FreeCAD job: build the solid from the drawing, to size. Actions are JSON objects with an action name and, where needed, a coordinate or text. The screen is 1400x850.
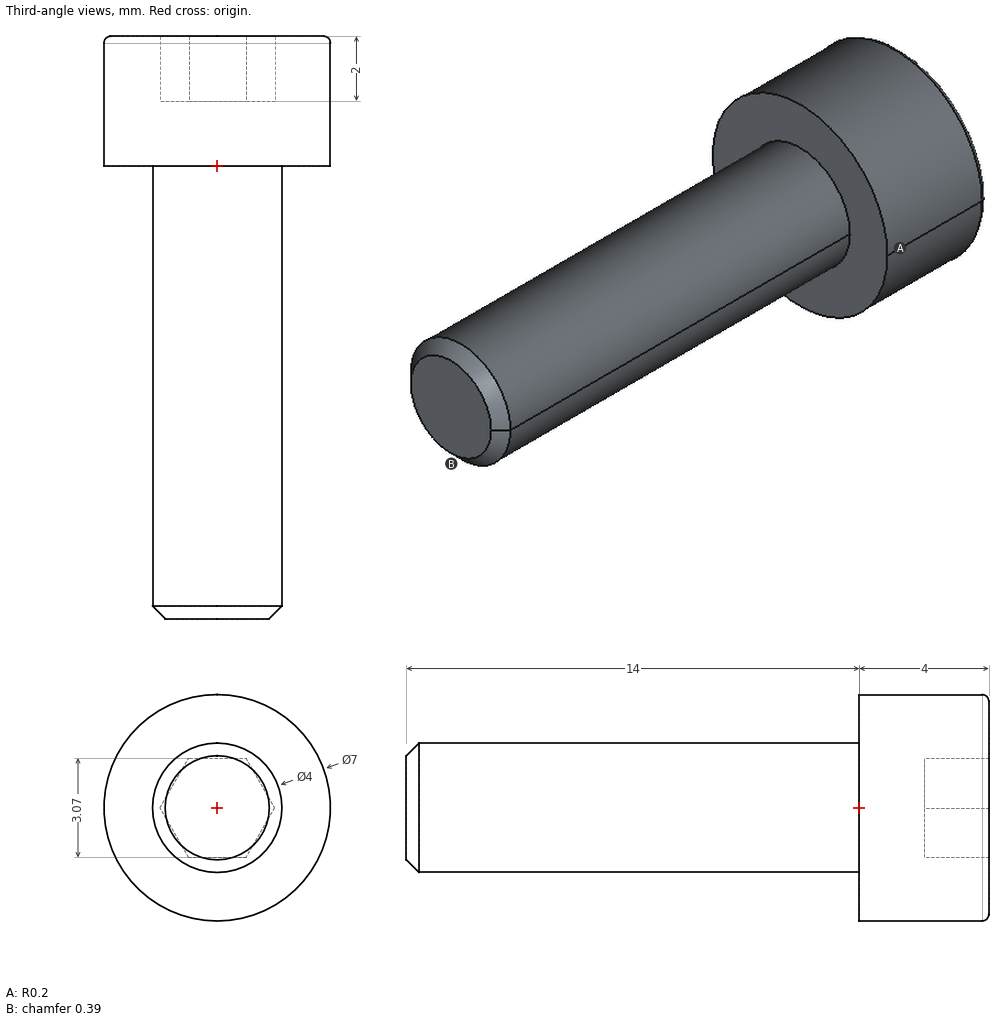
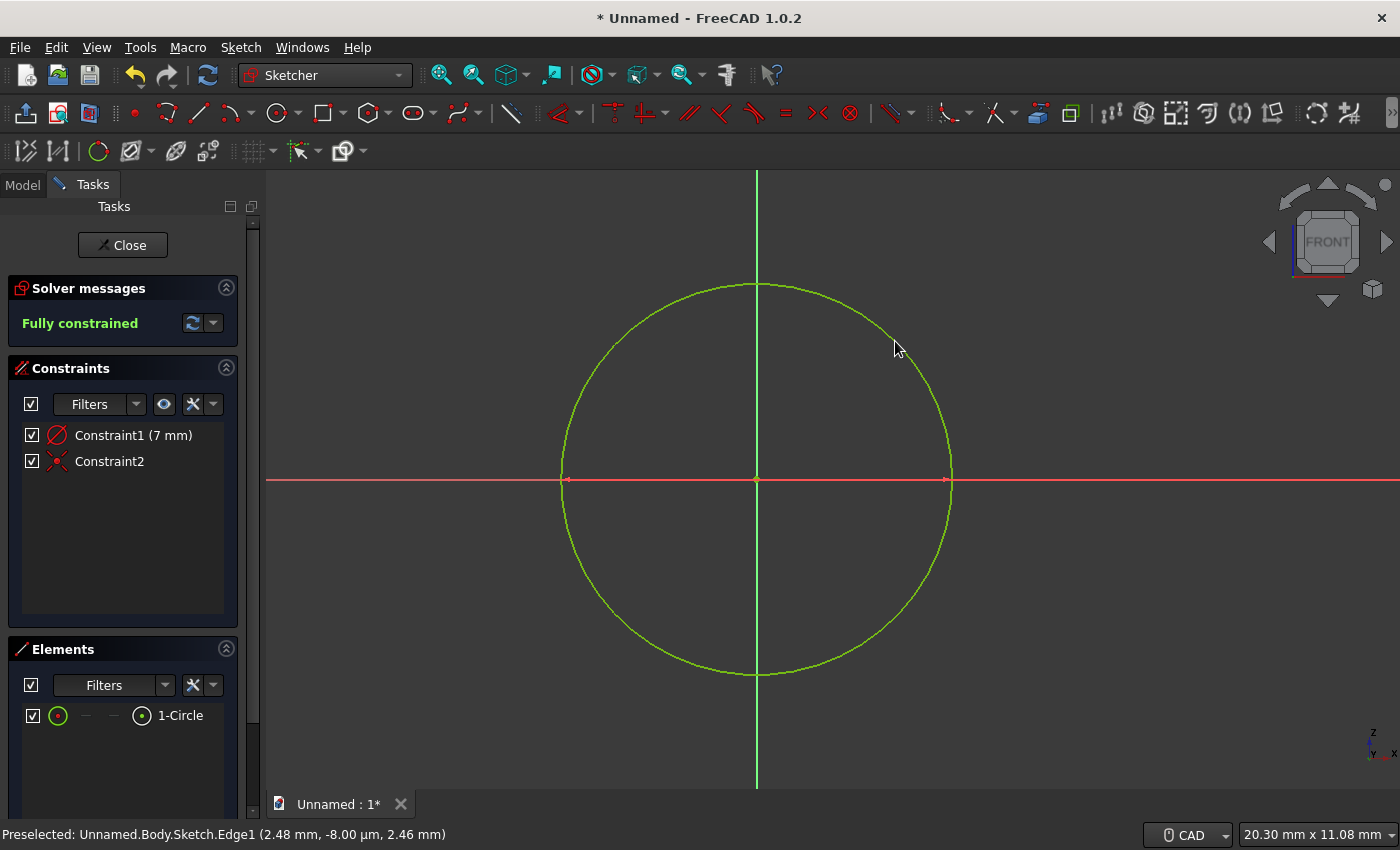
{"action": "left_click", "coordinate": [123, 245]}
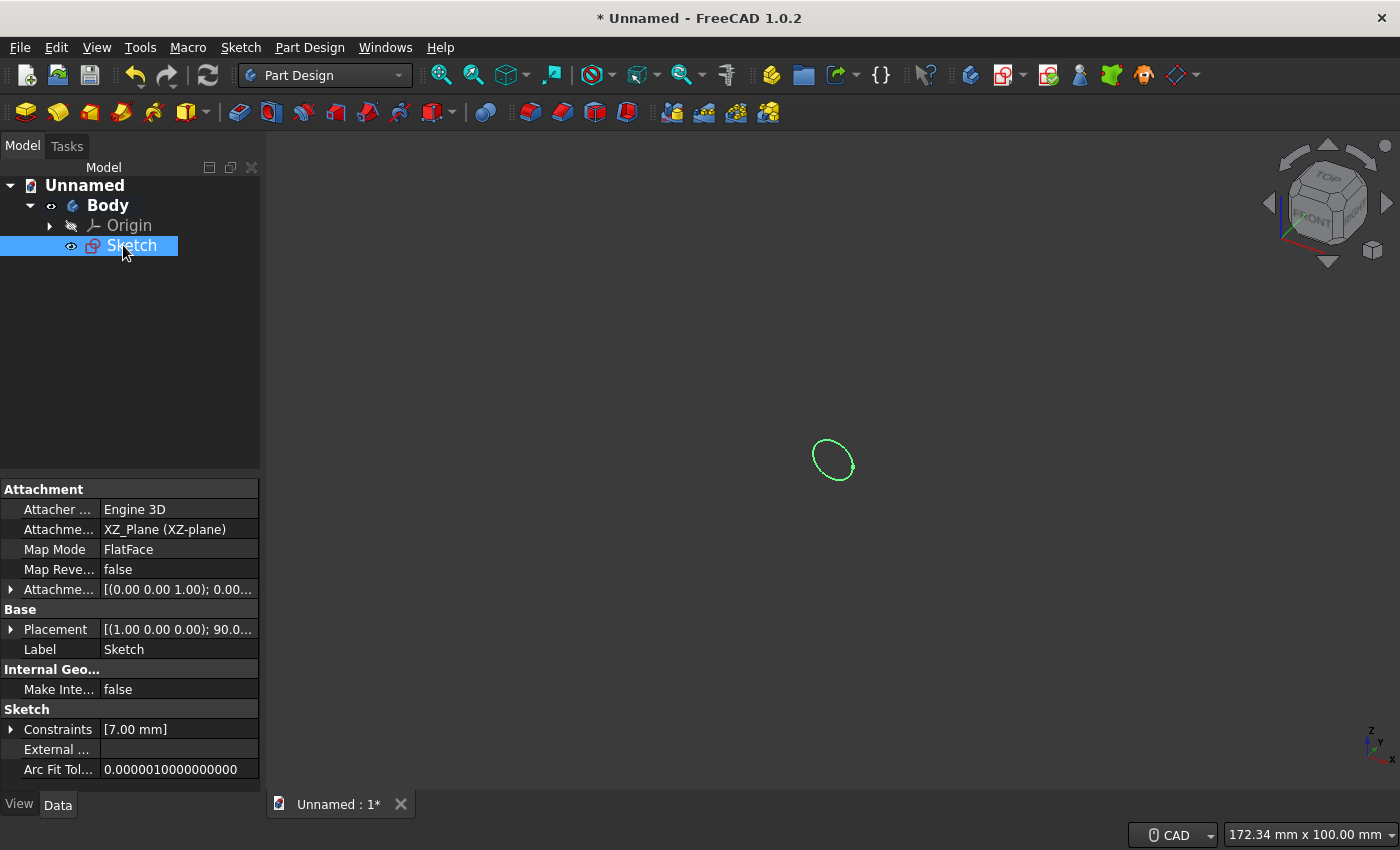
{"action": "left_click", "coordinate": [26, 112]}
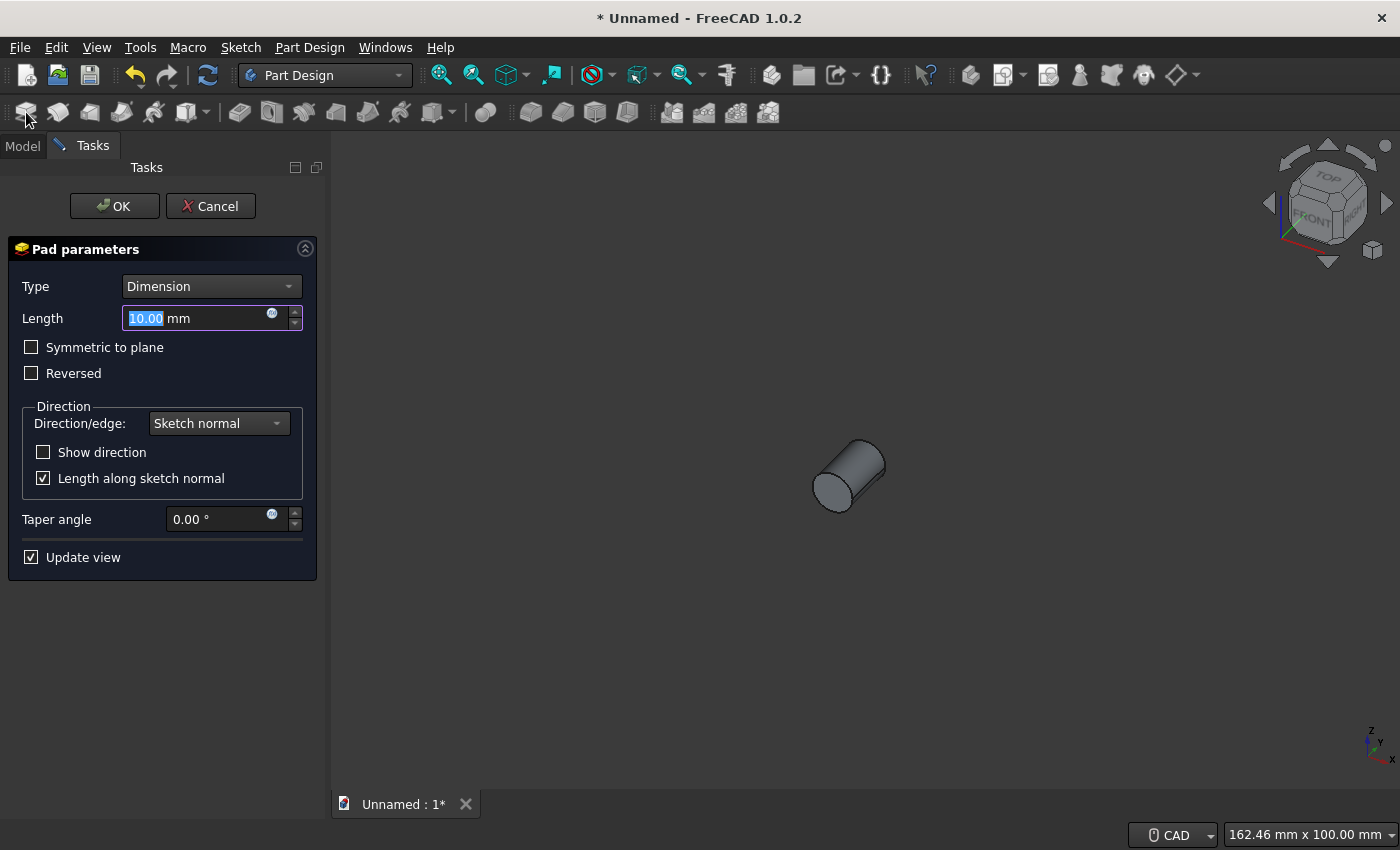
{"action": "type", "text": "4"}
{"action": "key", "text": "Tab"}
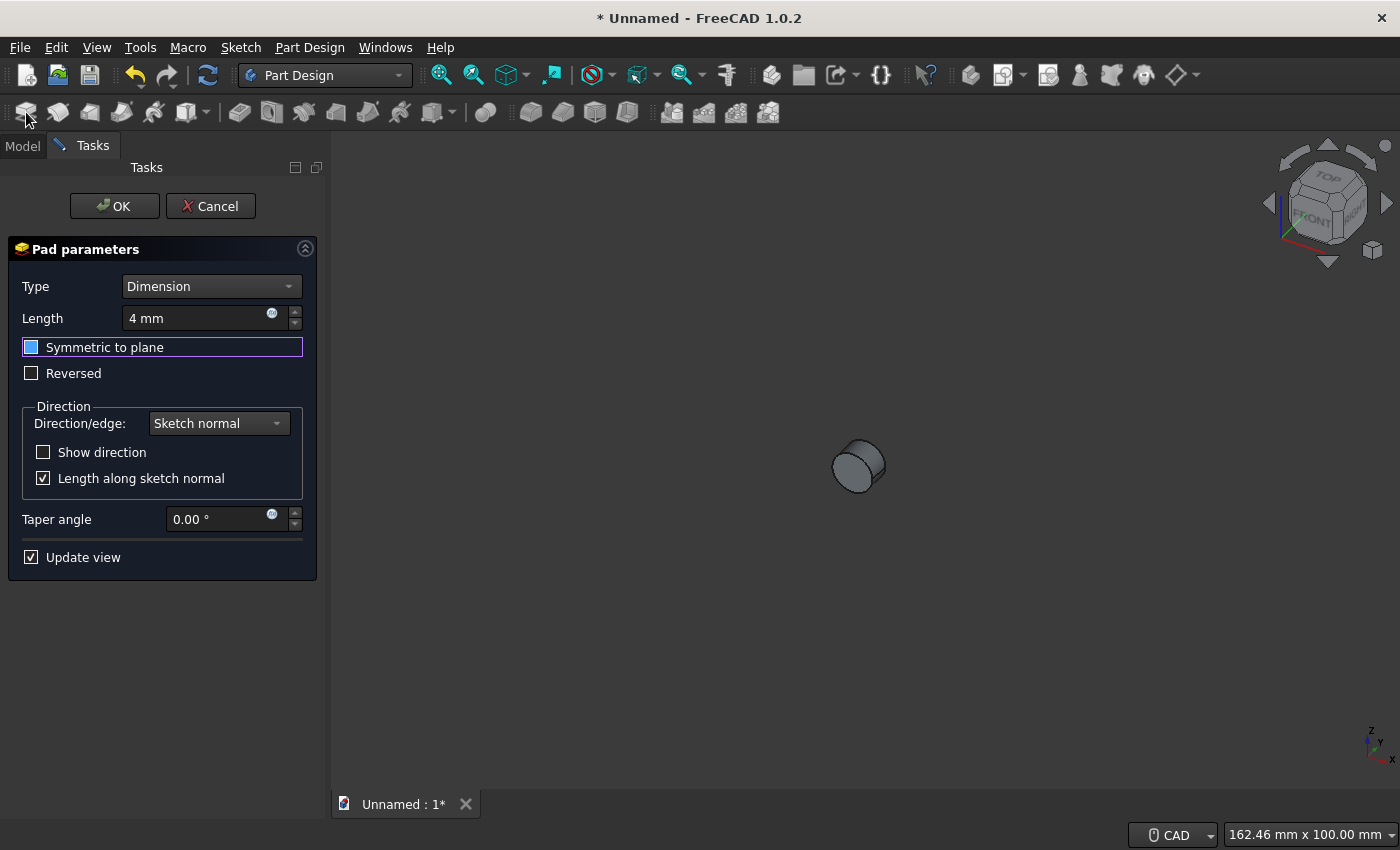
{"action": "left_click", "coordinate": [30, 373]}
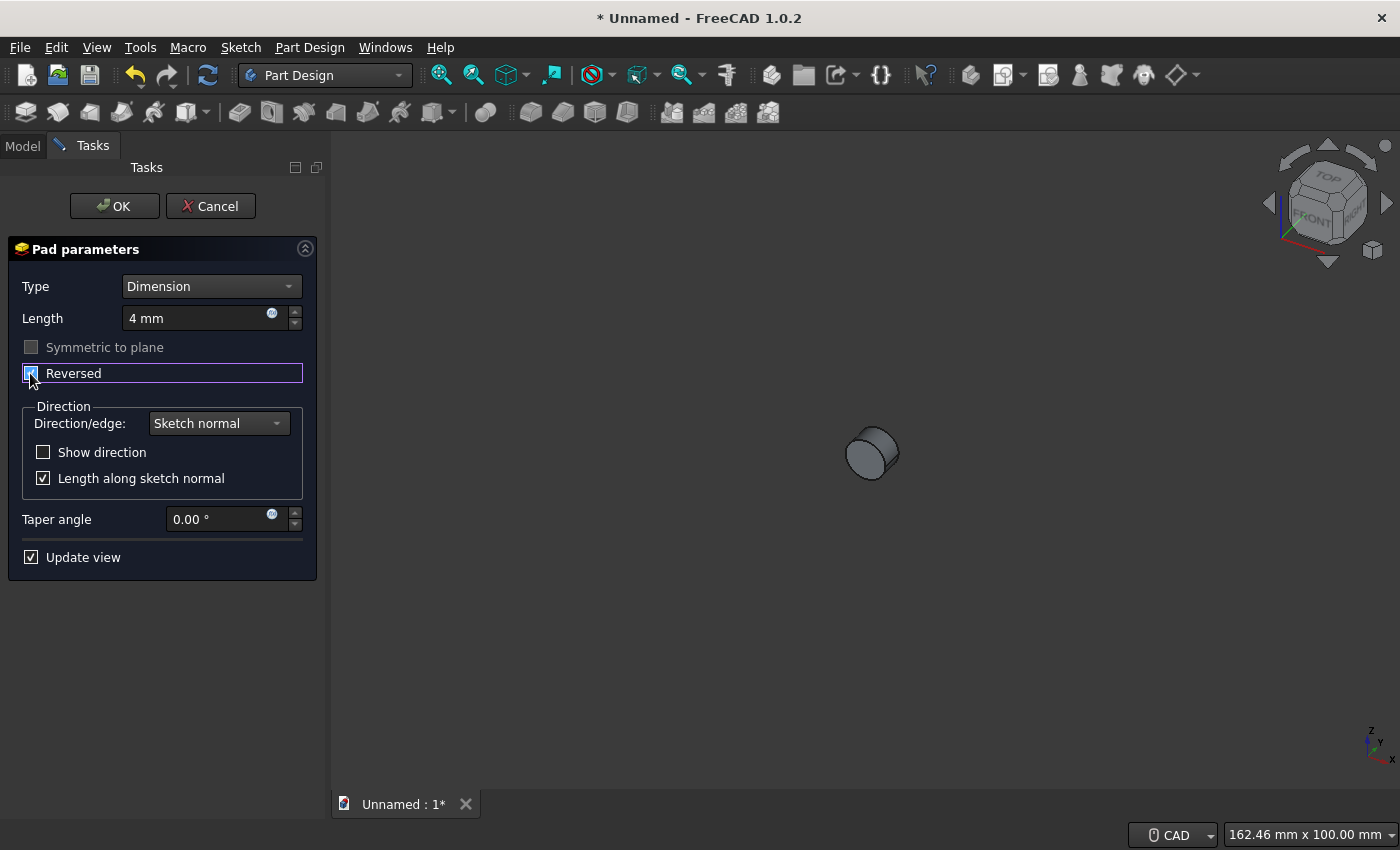
{"action": "left_click", "coordinate": [115, 206]}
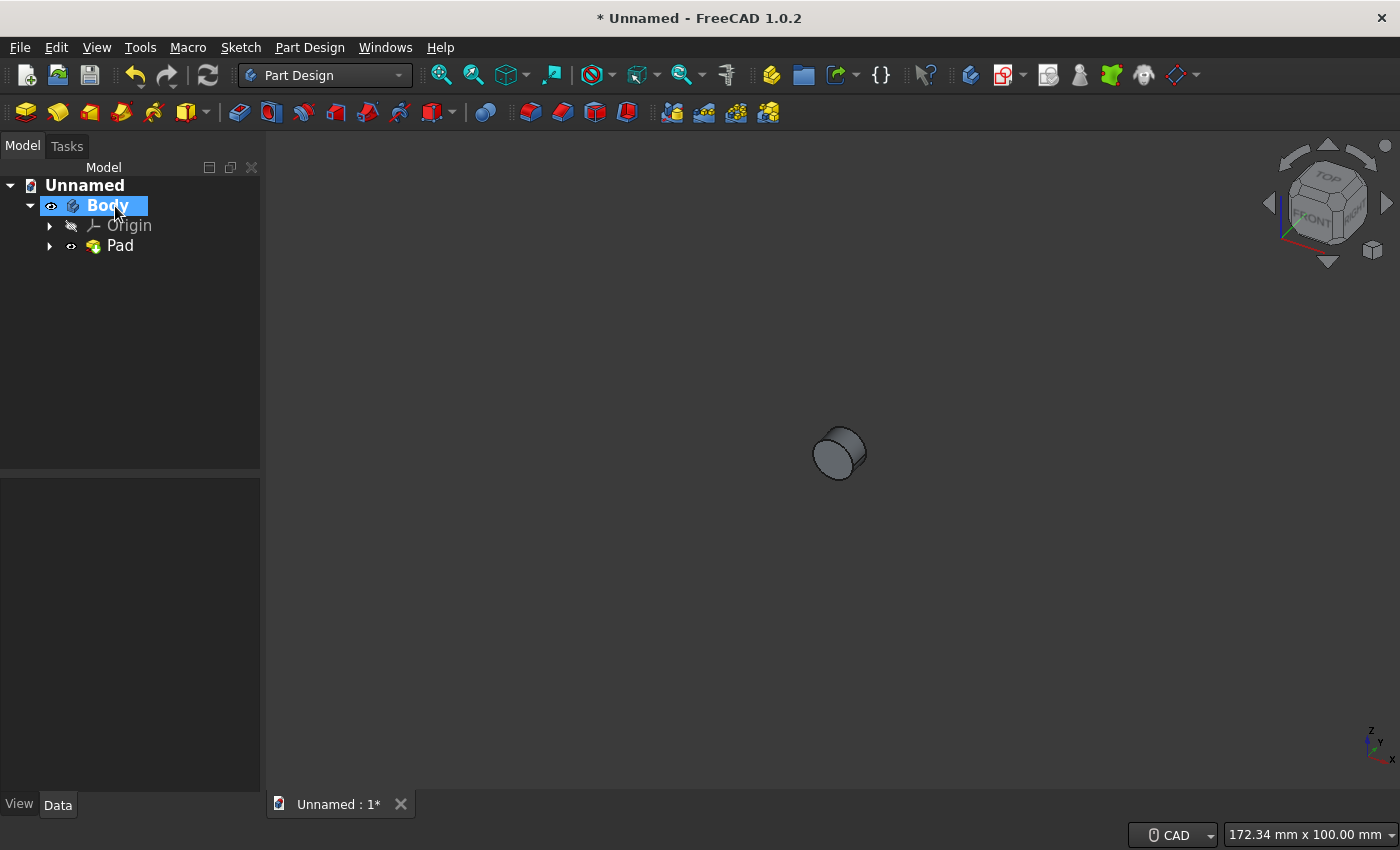
{"action": "left_click", "coordinate": [442, 76]}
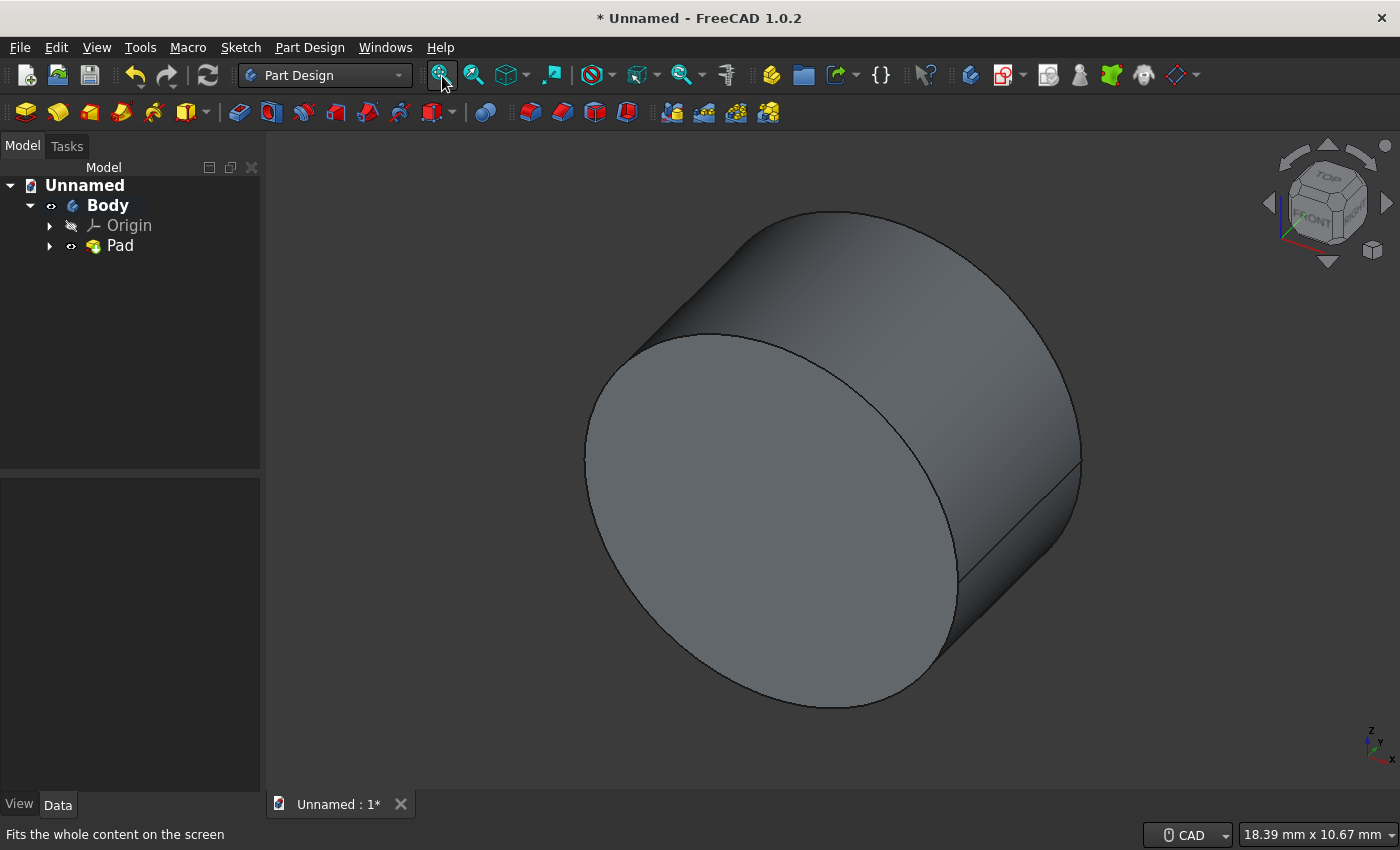
{"action": "key", "text": "4"}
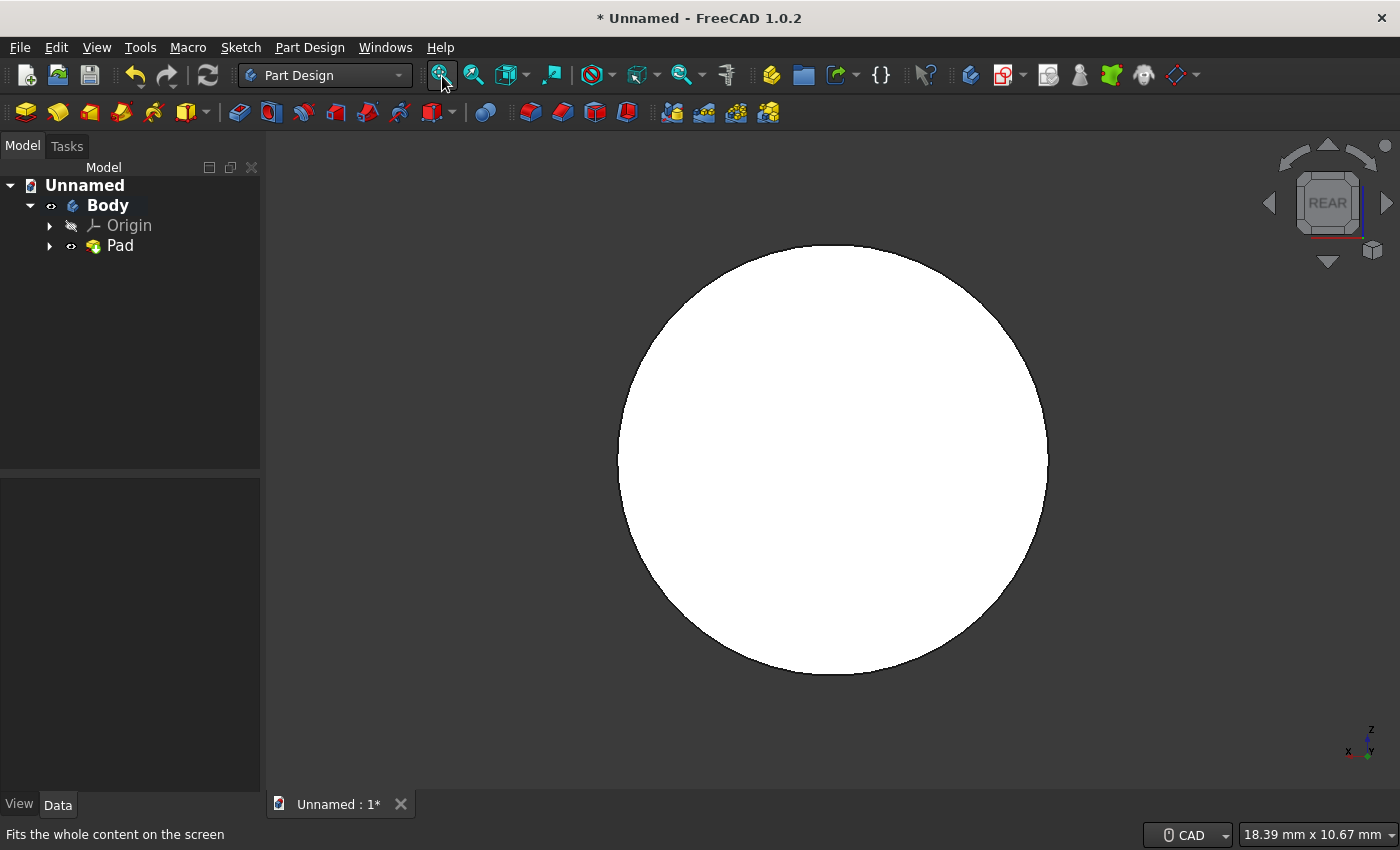
{"action": "left_click", "coordinate": [833, 459]}